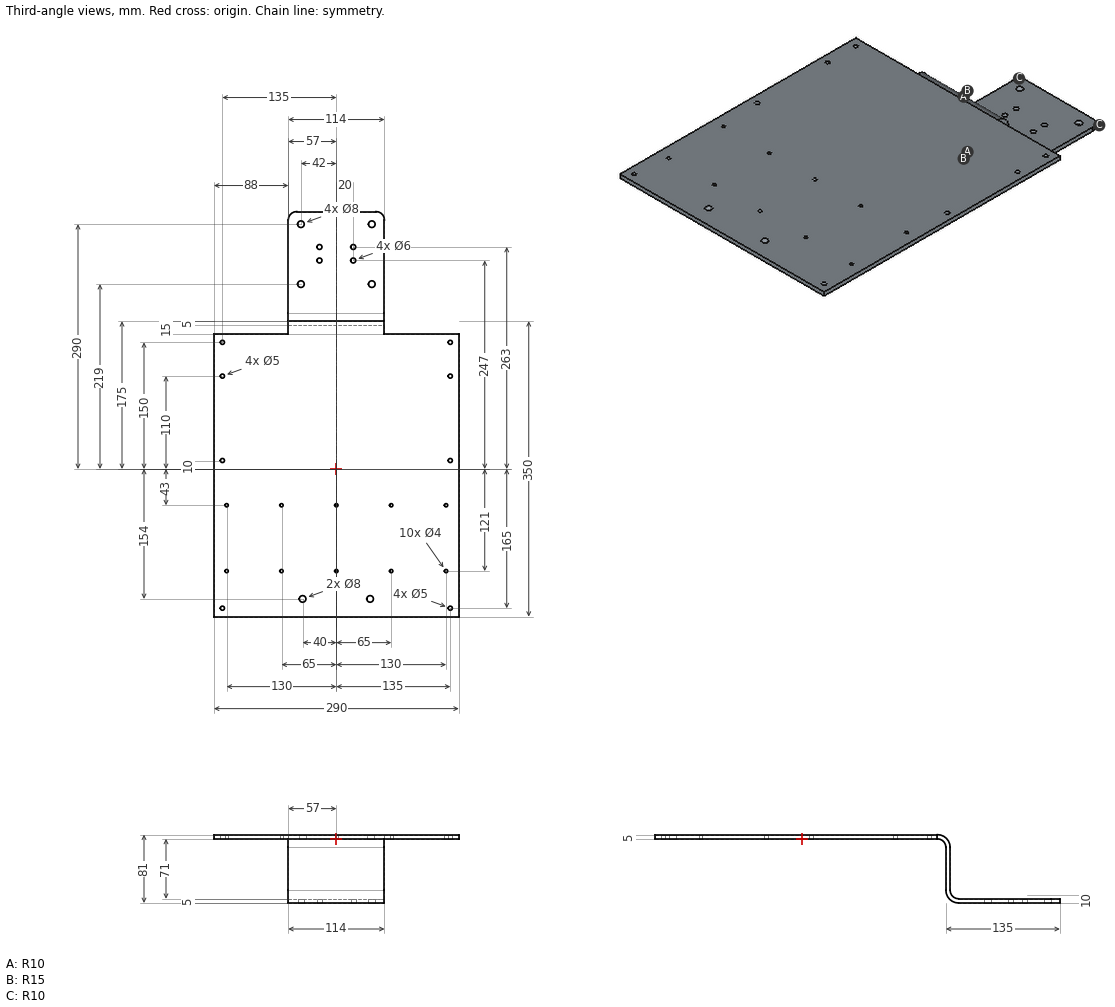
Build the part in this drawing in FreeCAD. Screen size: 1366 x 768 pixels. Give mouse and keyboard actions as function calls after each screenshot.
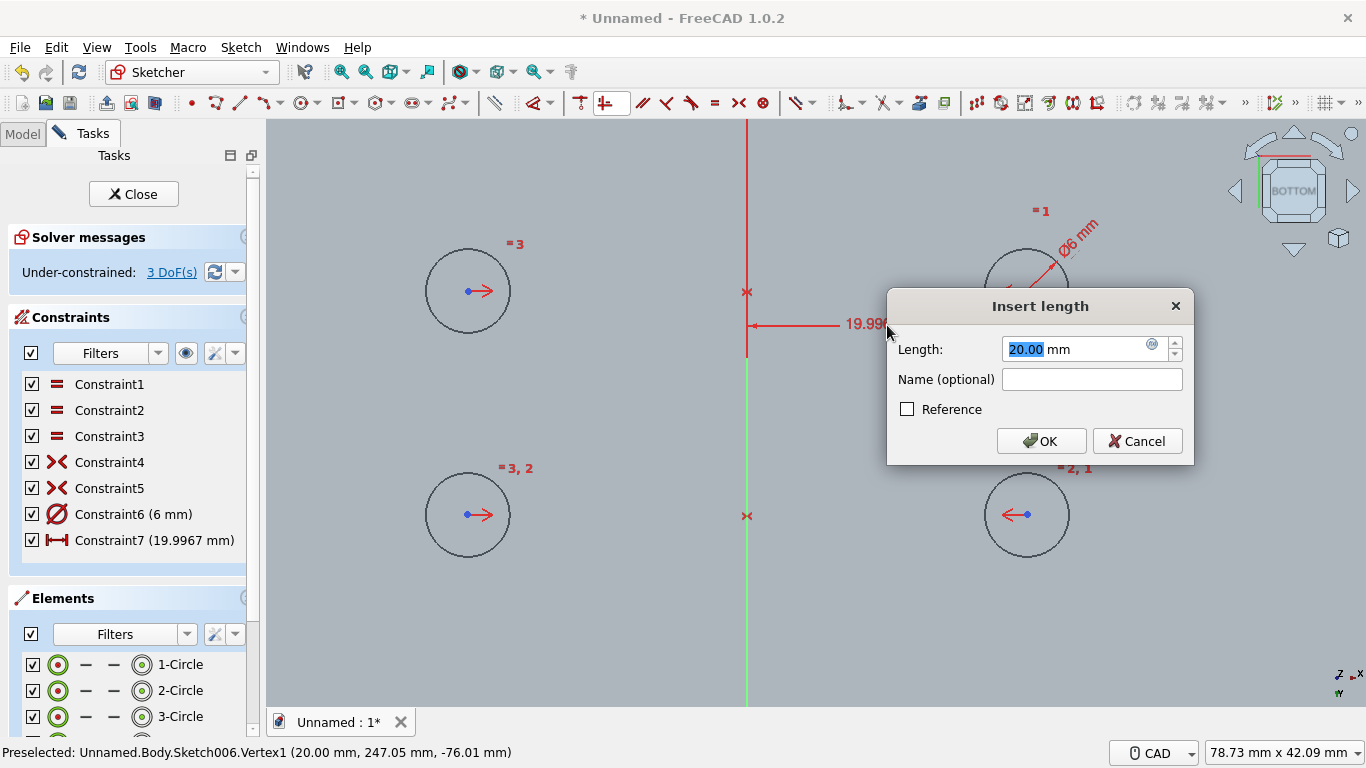
text(20)
key(Return)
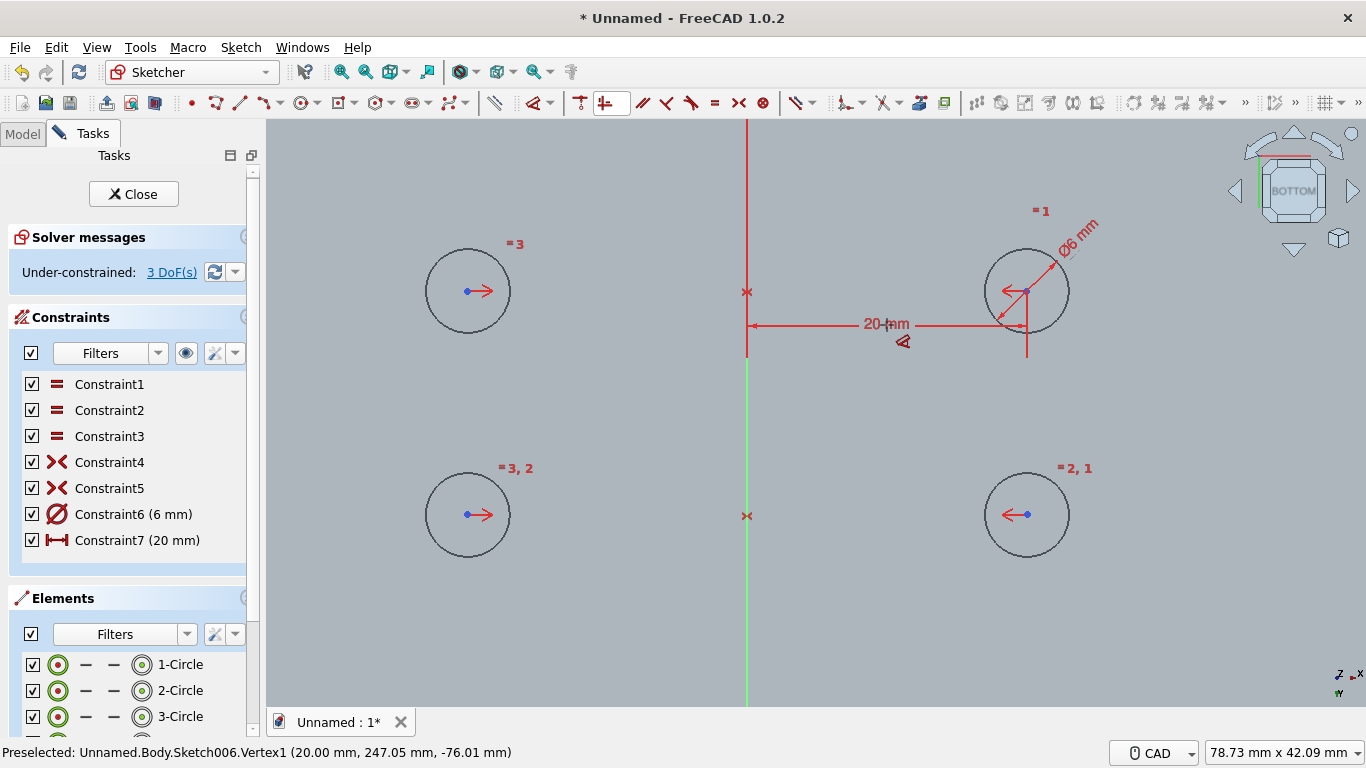
click(1027, 515)
click(887, 549)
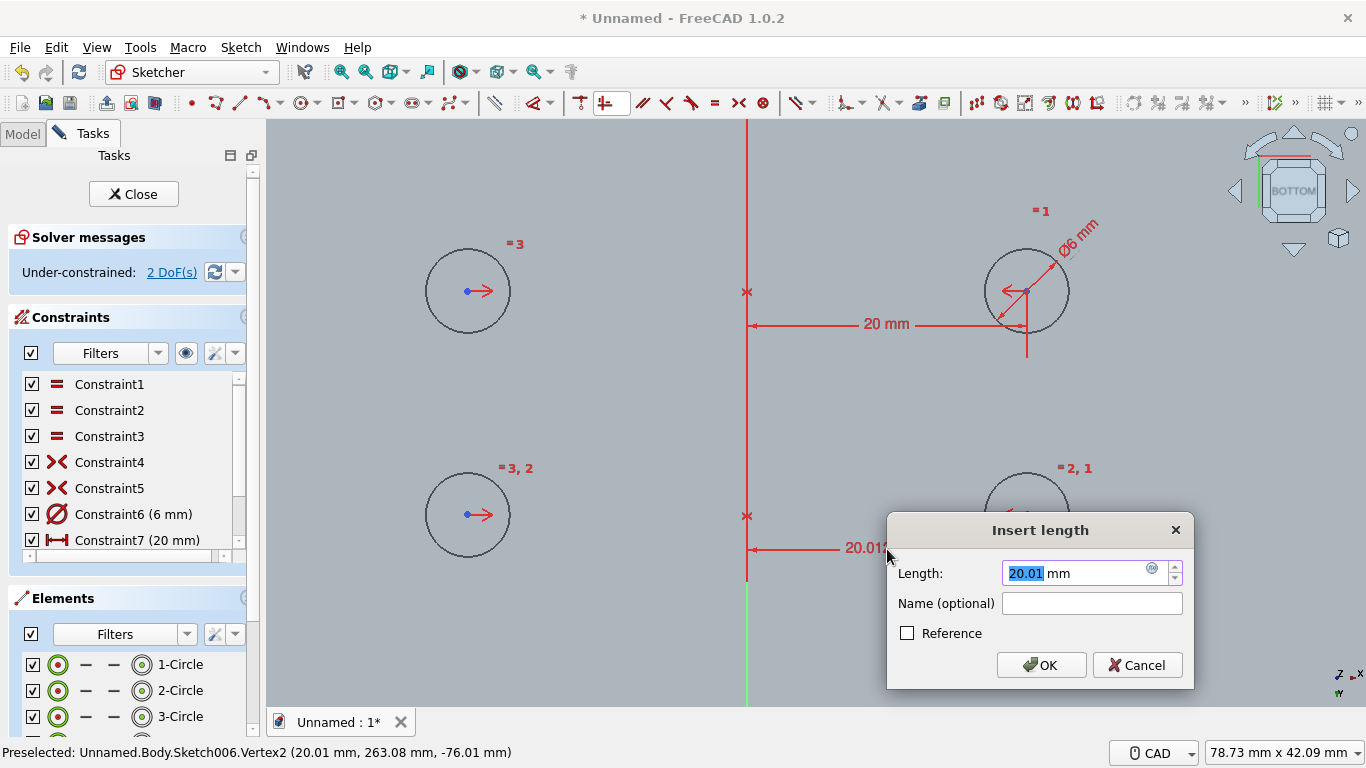
text(20)
key(Return)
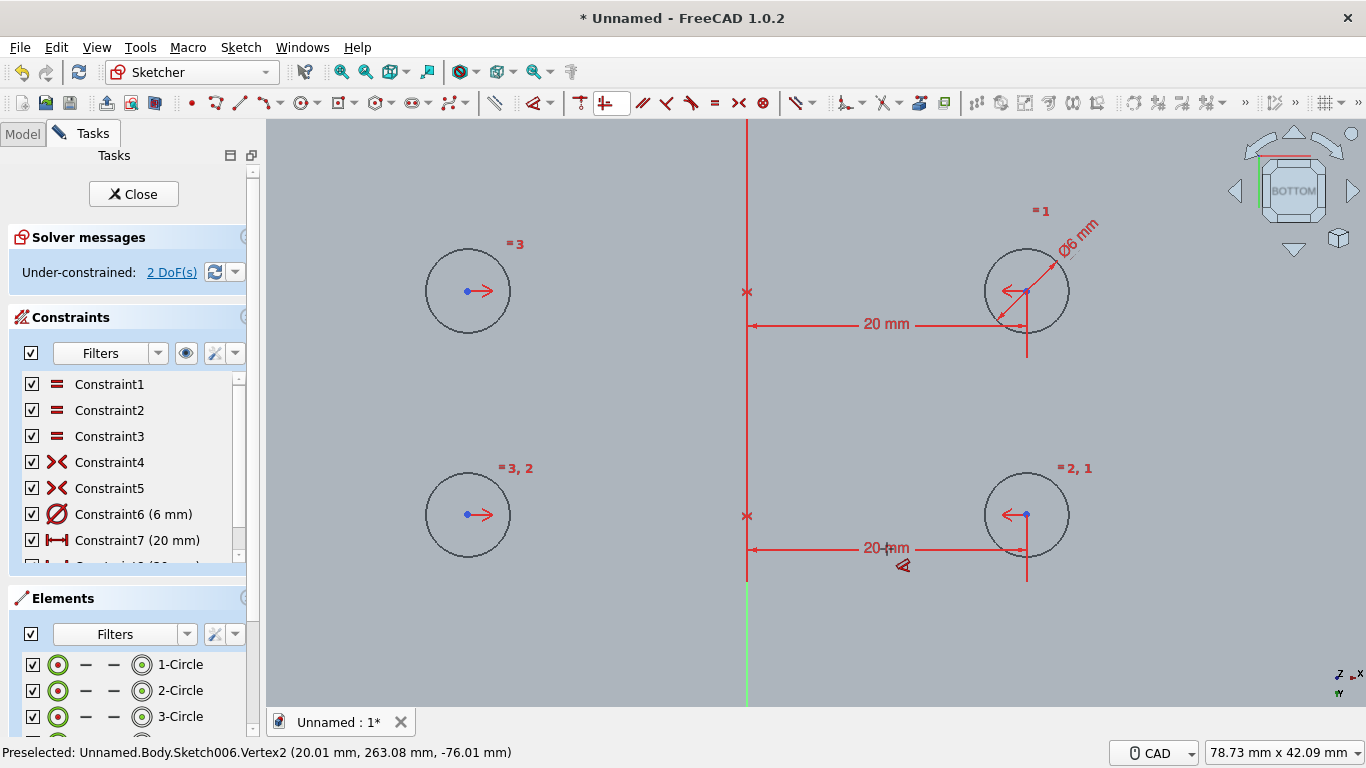
click(1027, 291)
click(1061, 219)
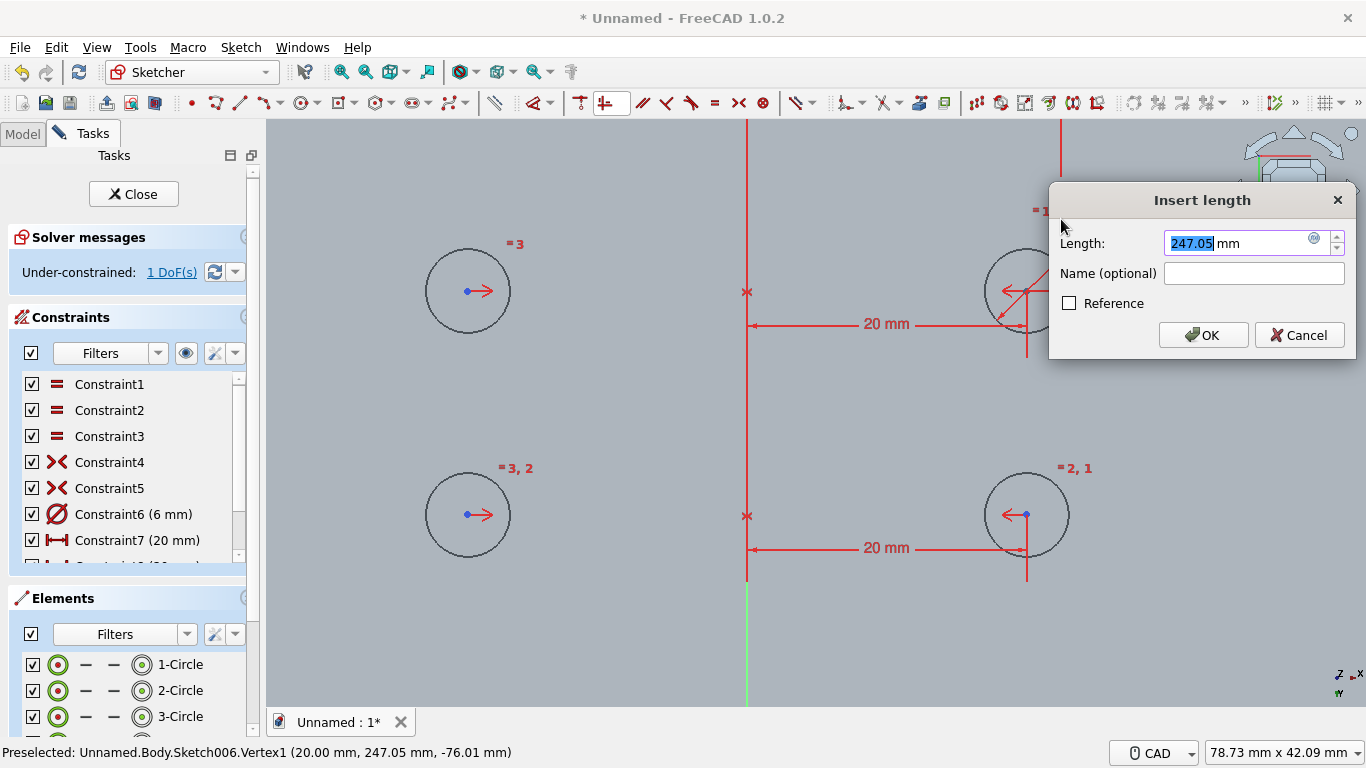
text(247)
key(Return)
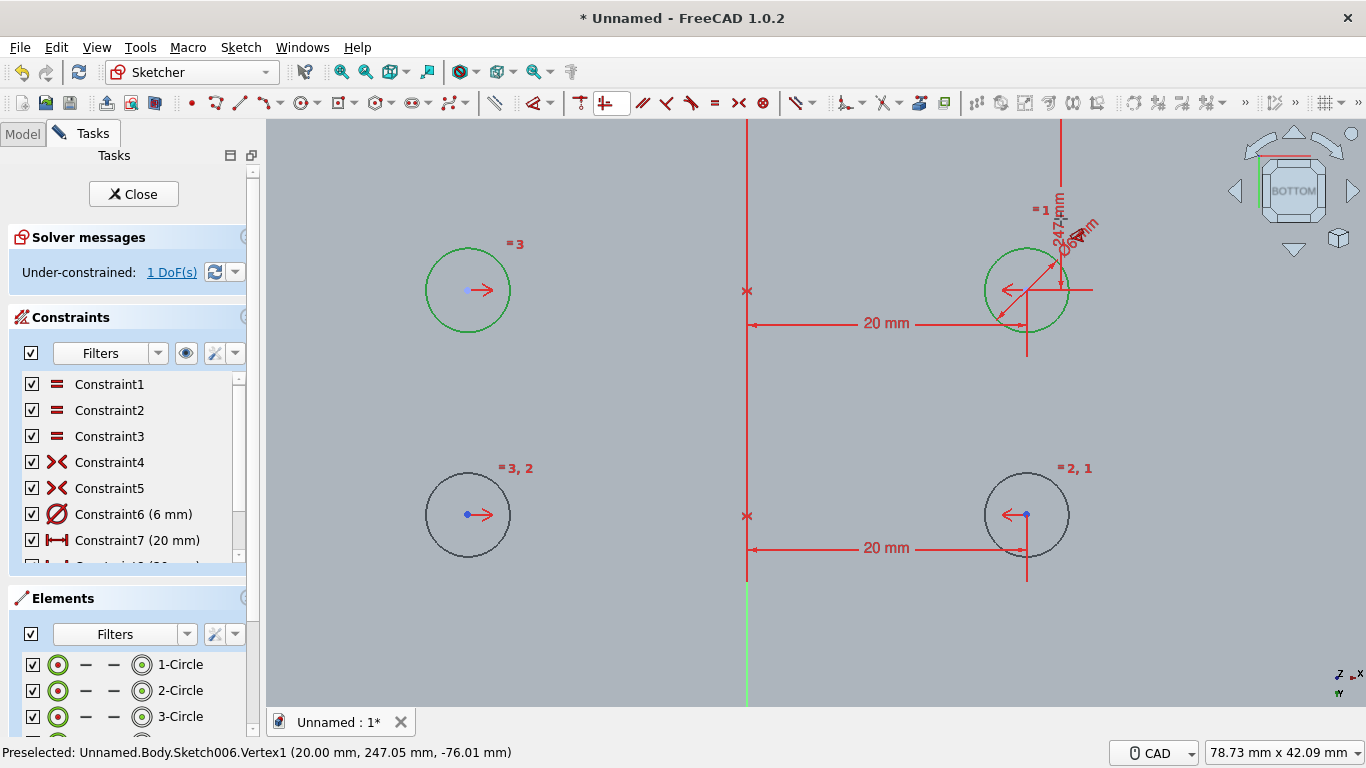
click(1027, 515)
click(1061, 416)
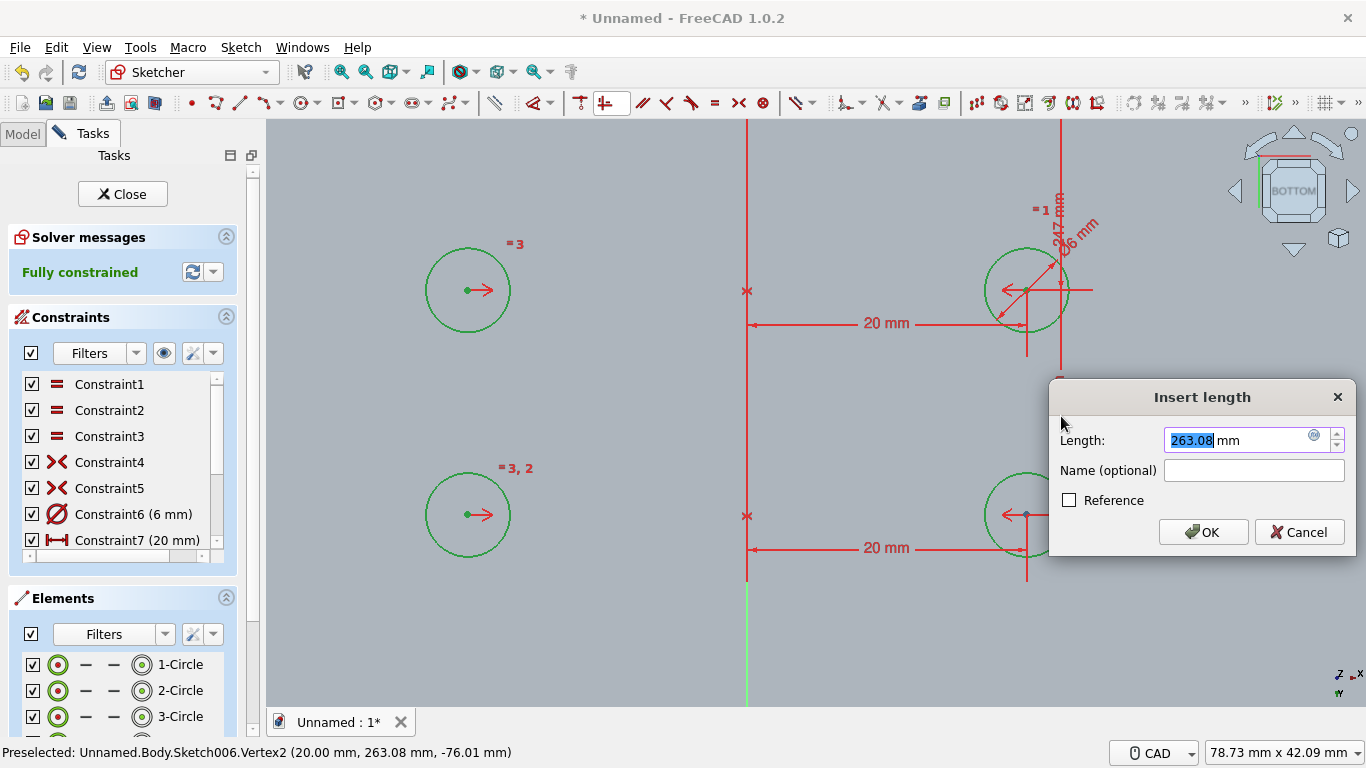
text(263)
key(Return)
key(Escape)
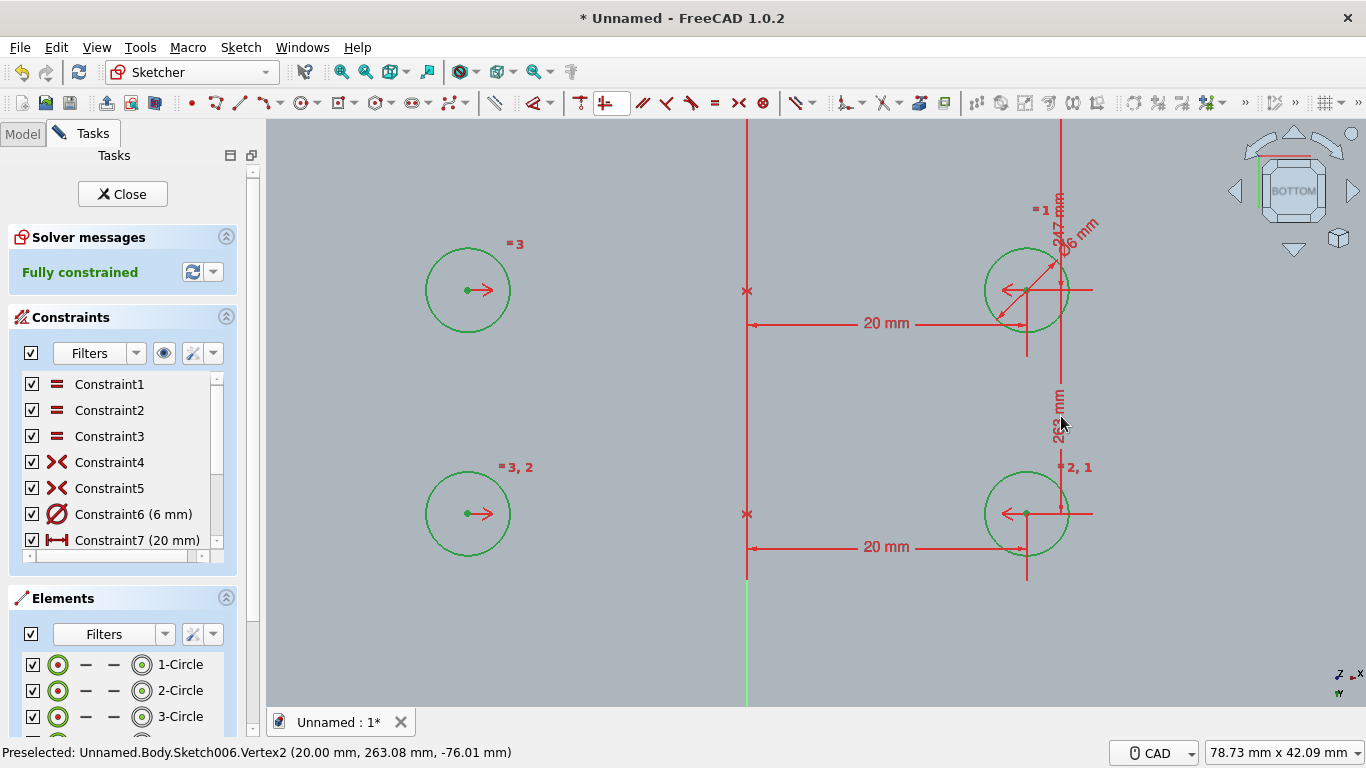
click(123, 194)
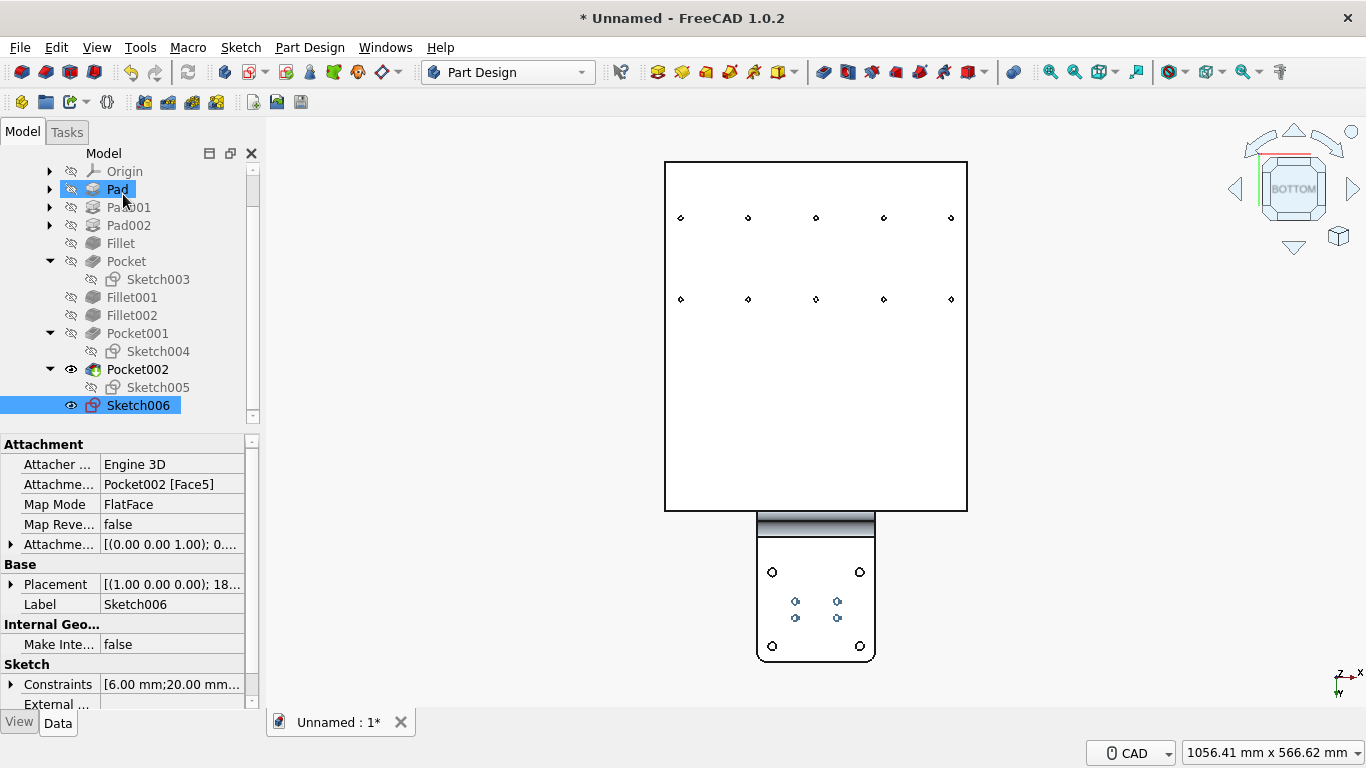
click(824, 72)